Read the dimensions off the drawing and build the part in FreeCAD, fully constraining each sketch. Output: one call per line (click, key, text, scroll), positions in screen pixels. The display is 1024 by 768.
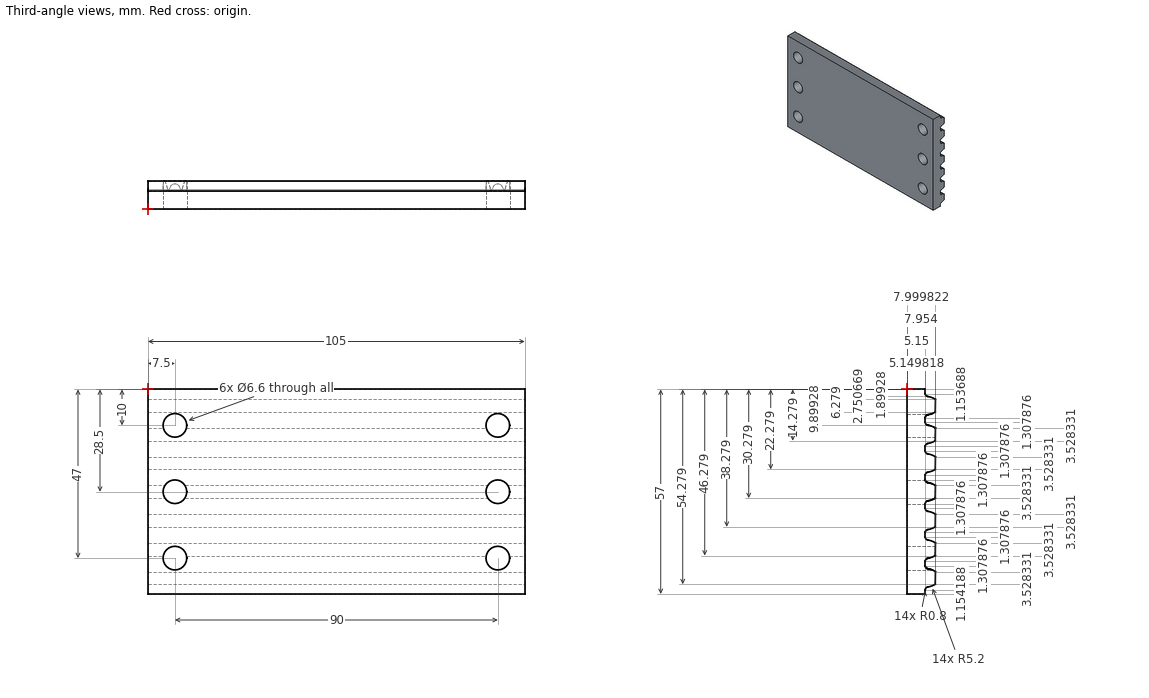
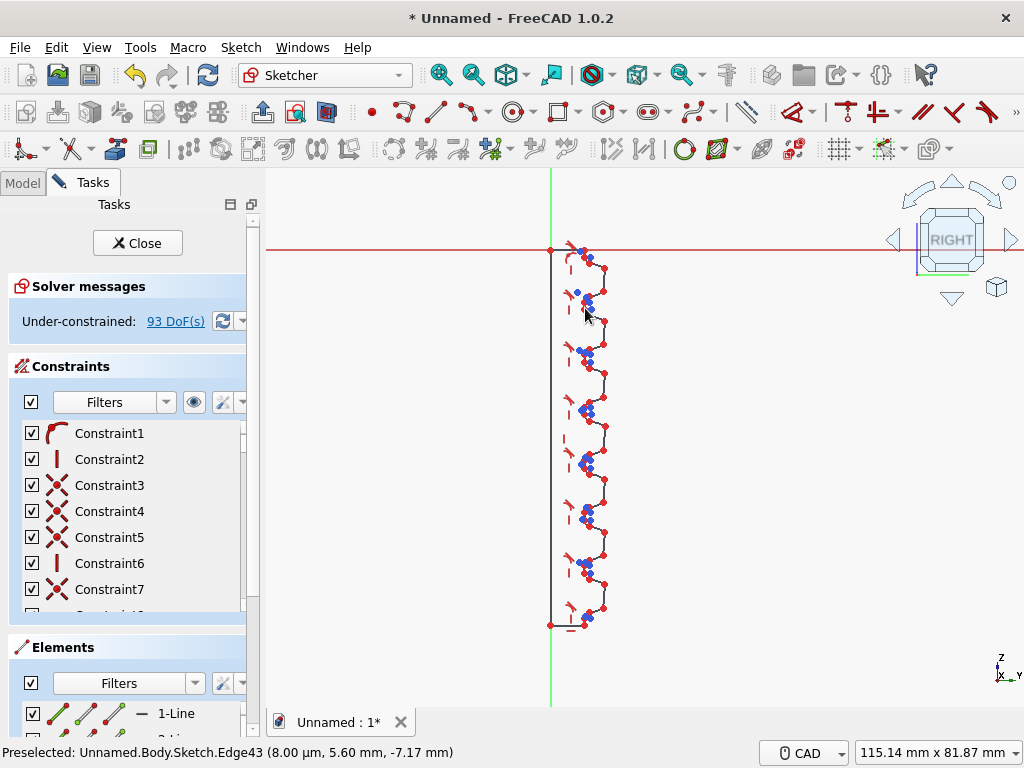
scroll(587, 614, up, 9)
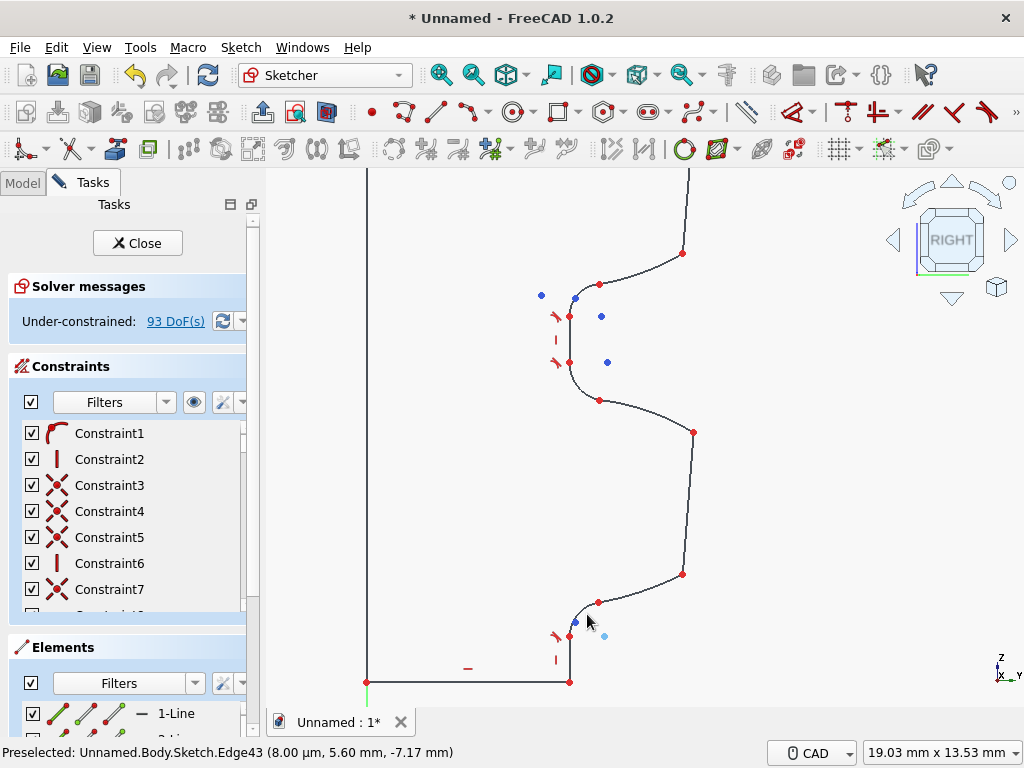
click(585, 608)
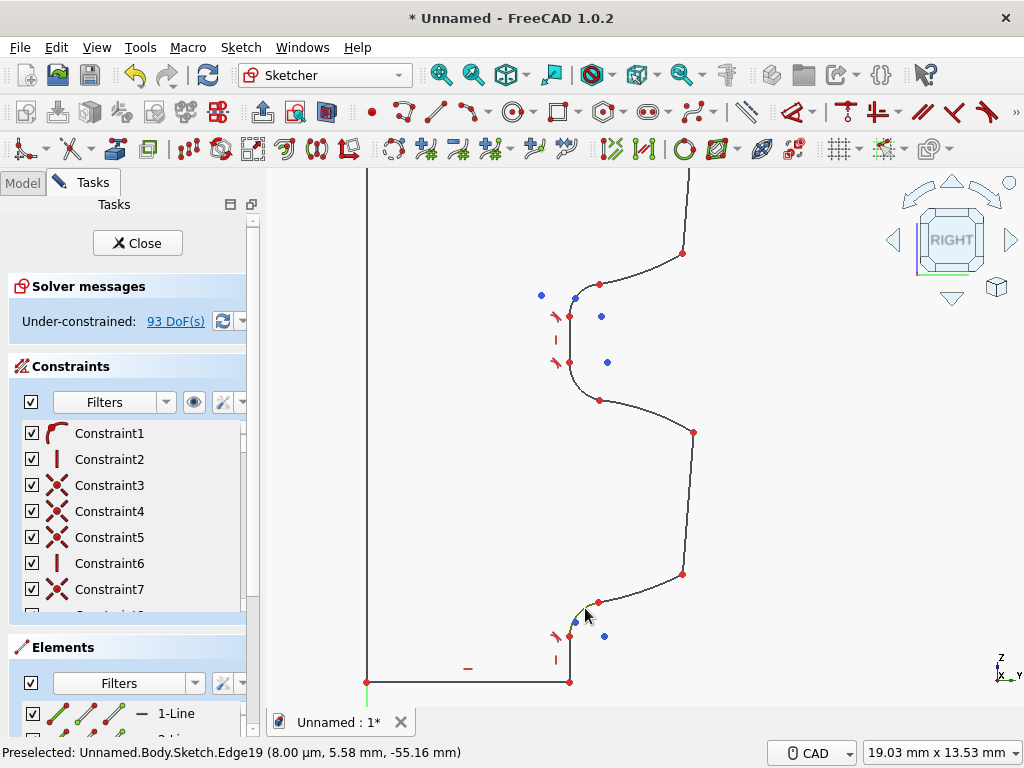
click(625, 597)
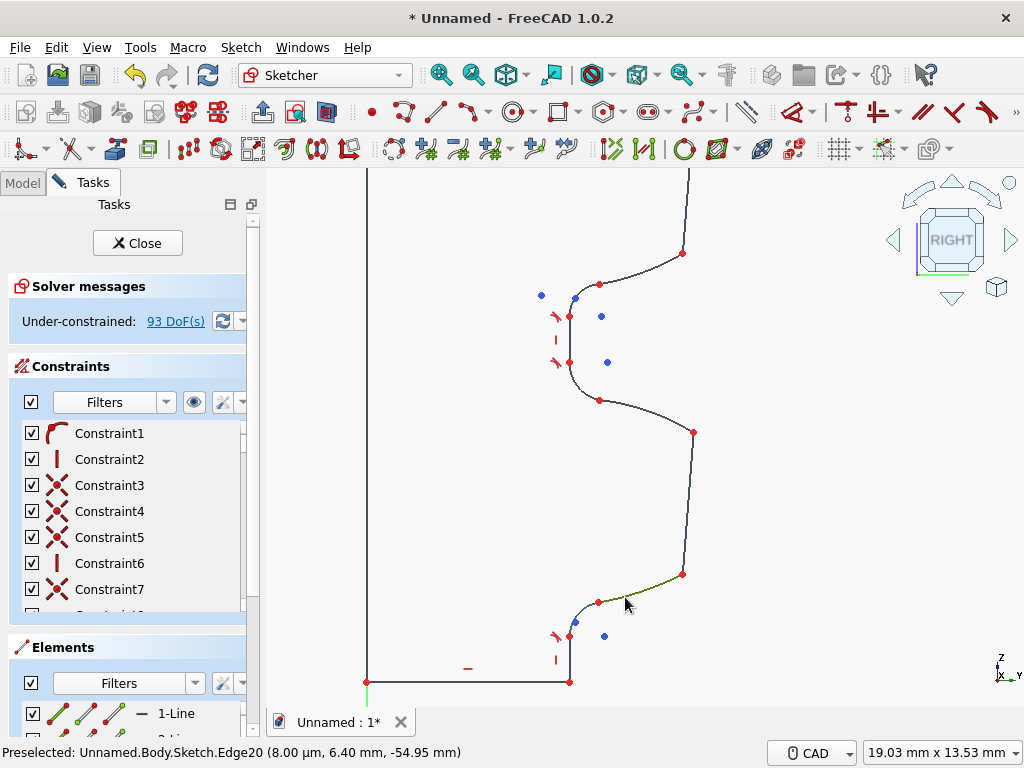
click(988, 112)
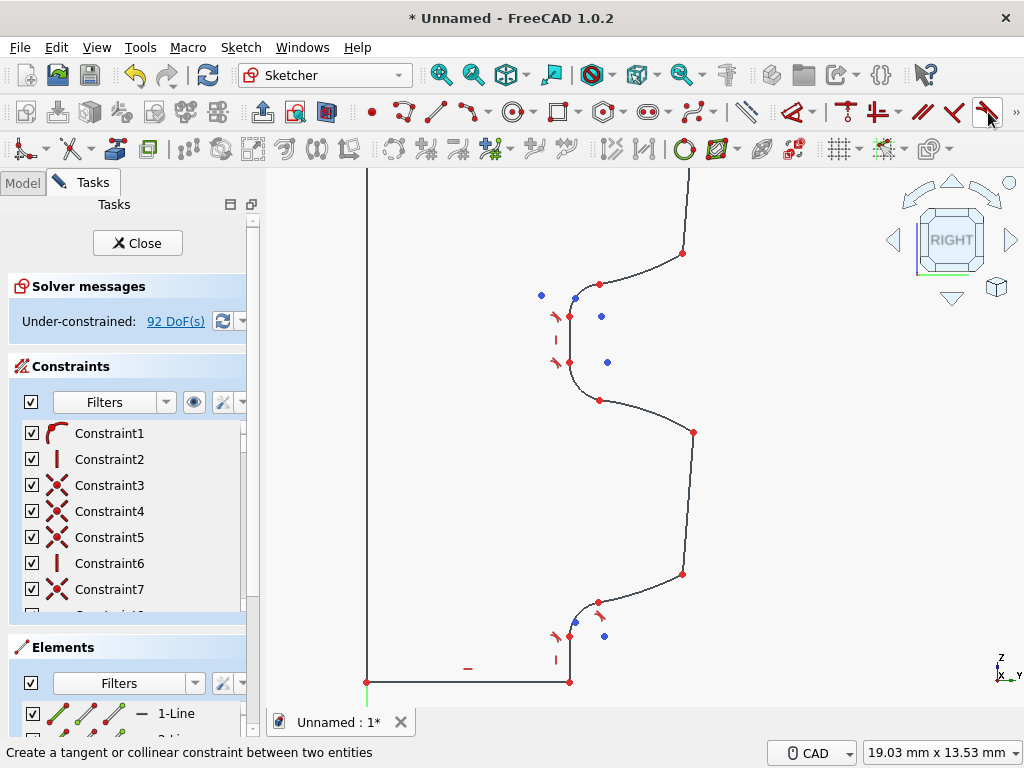
click(667, 419)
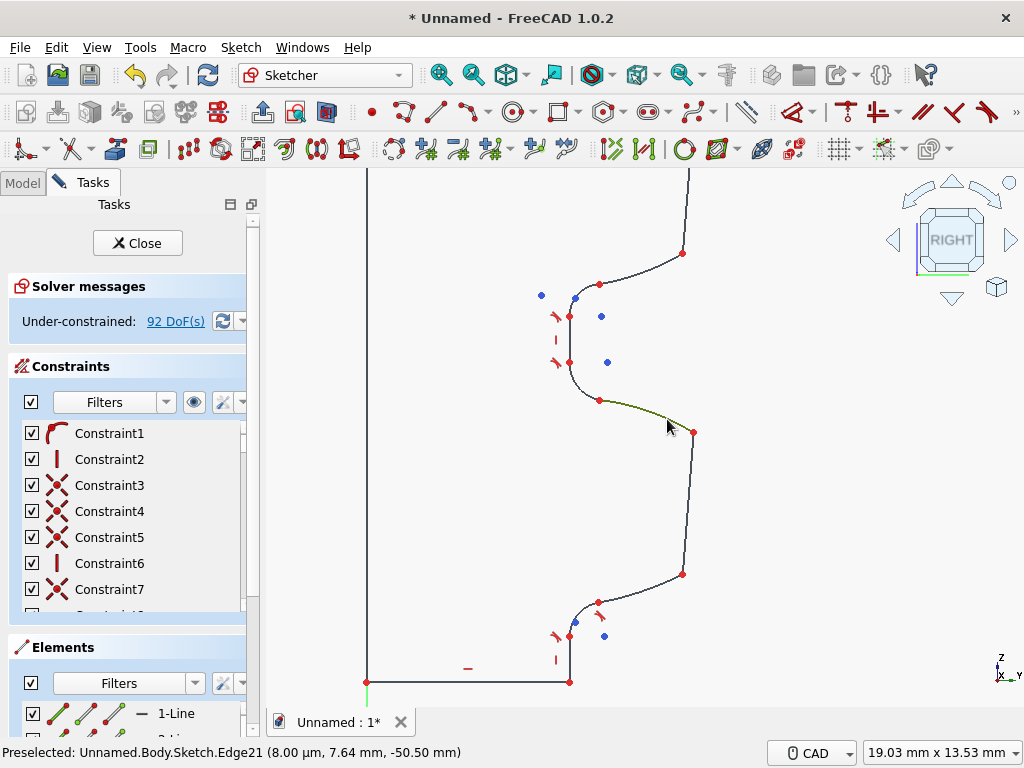
click(573, 378)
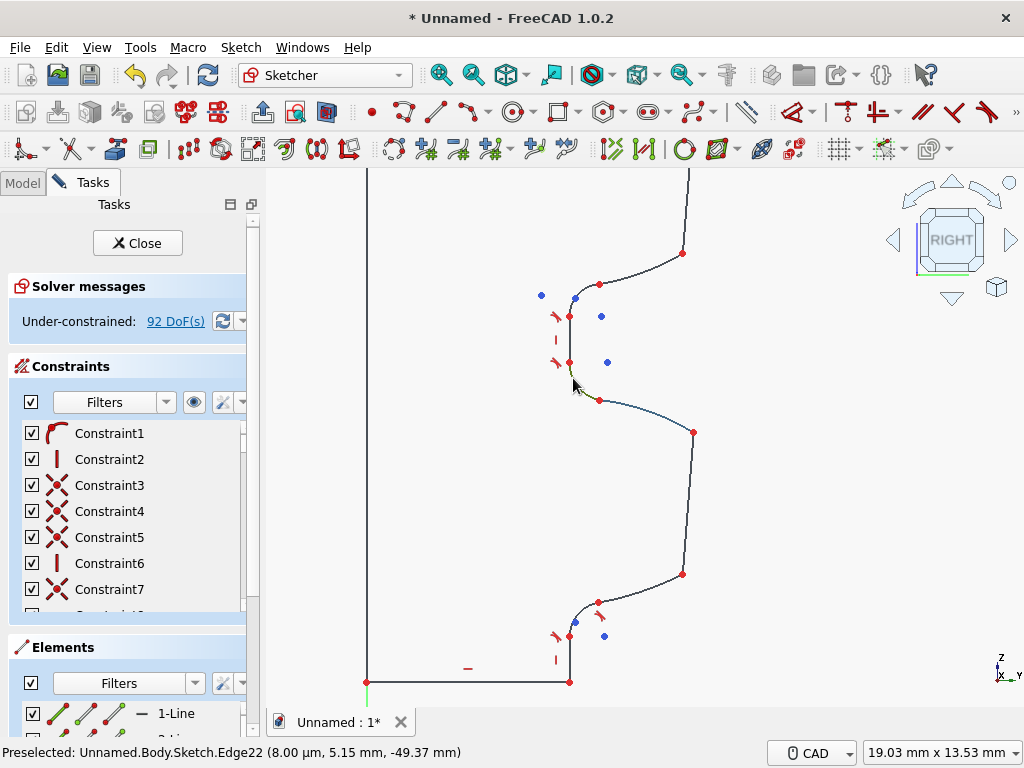
click(988, 112)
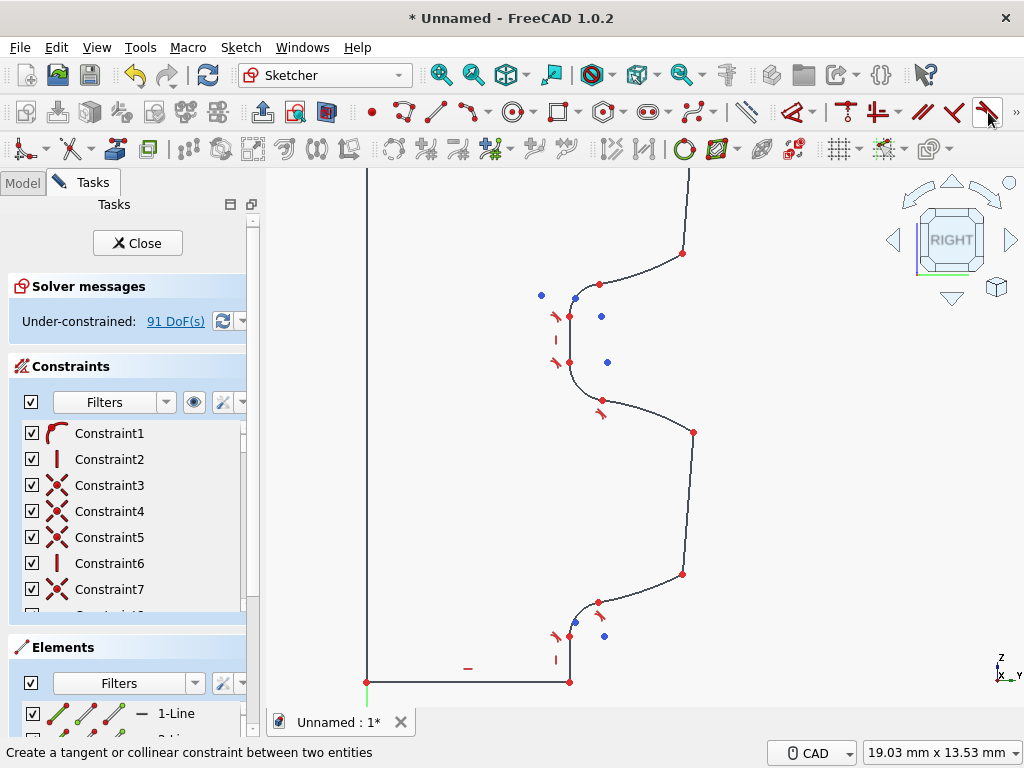
click(586, 288)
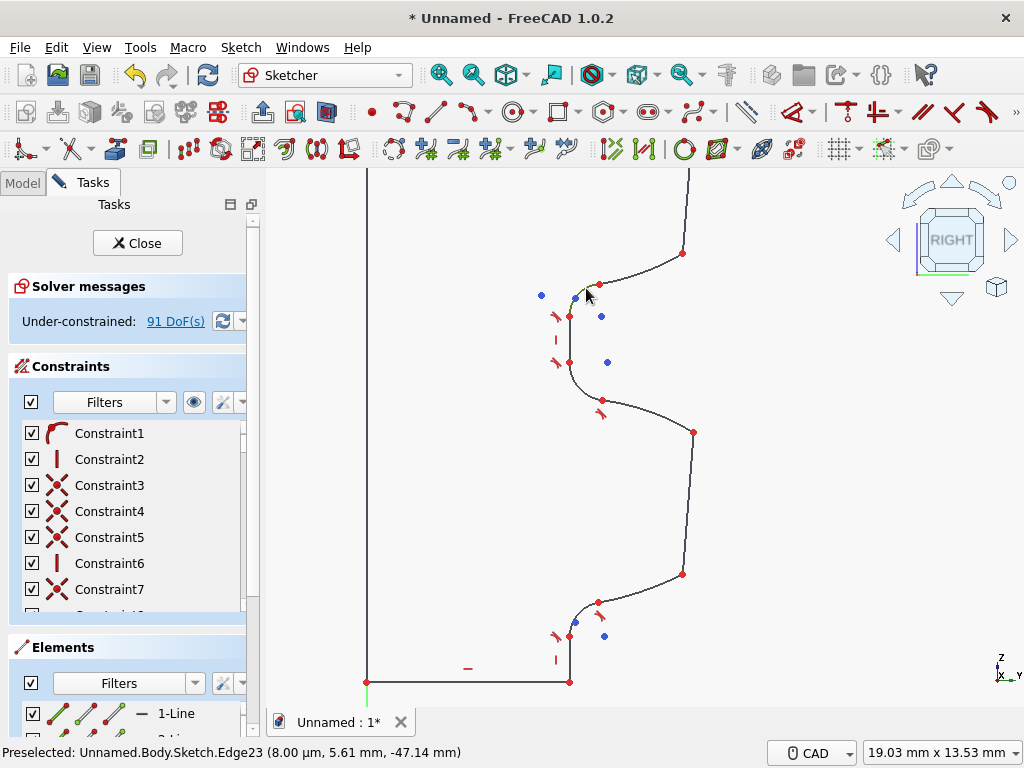
click(626, 278)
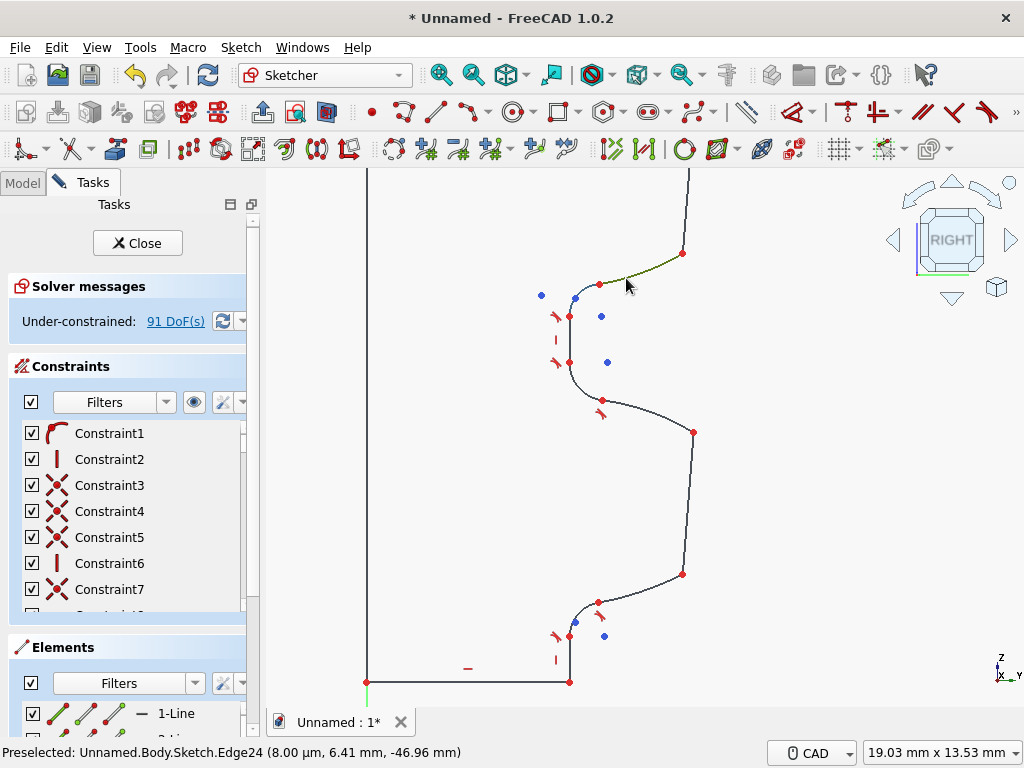
click(988, 112)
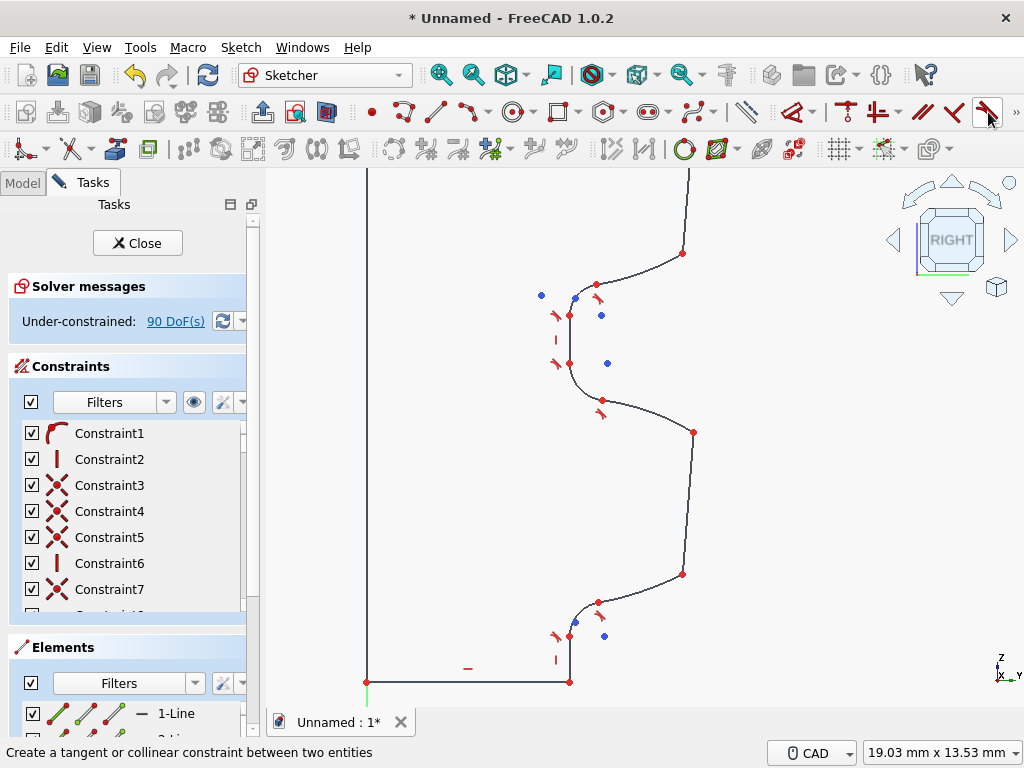
scroll(587, 614, down, 9)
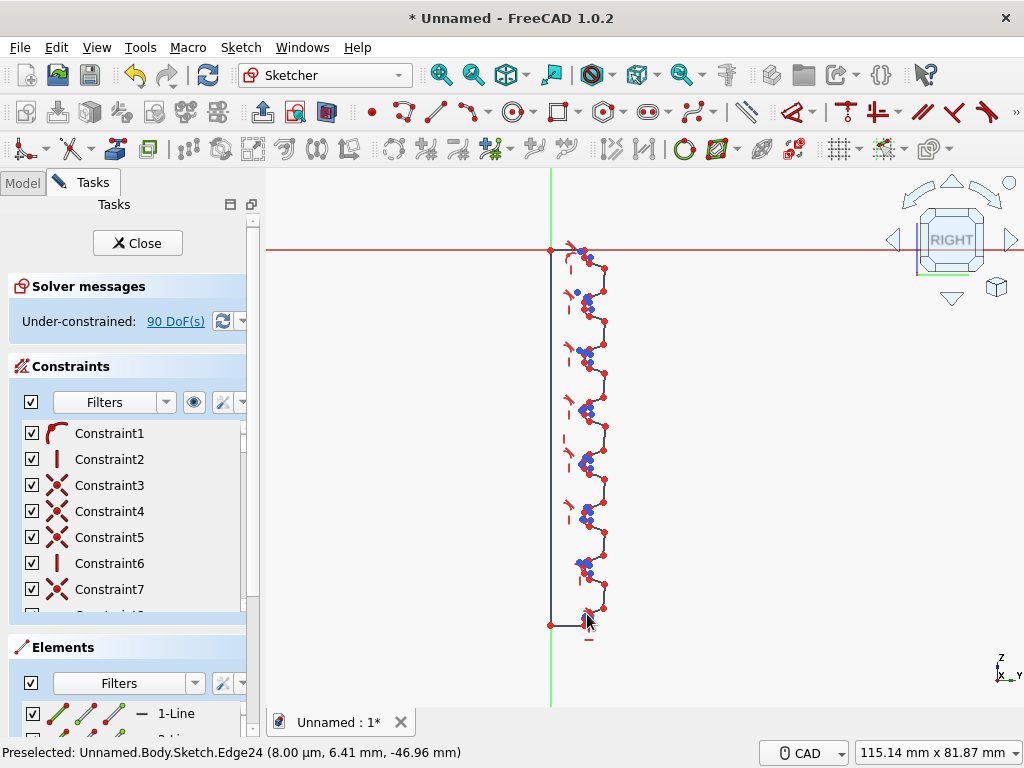
scroll(601, 530, up, 6)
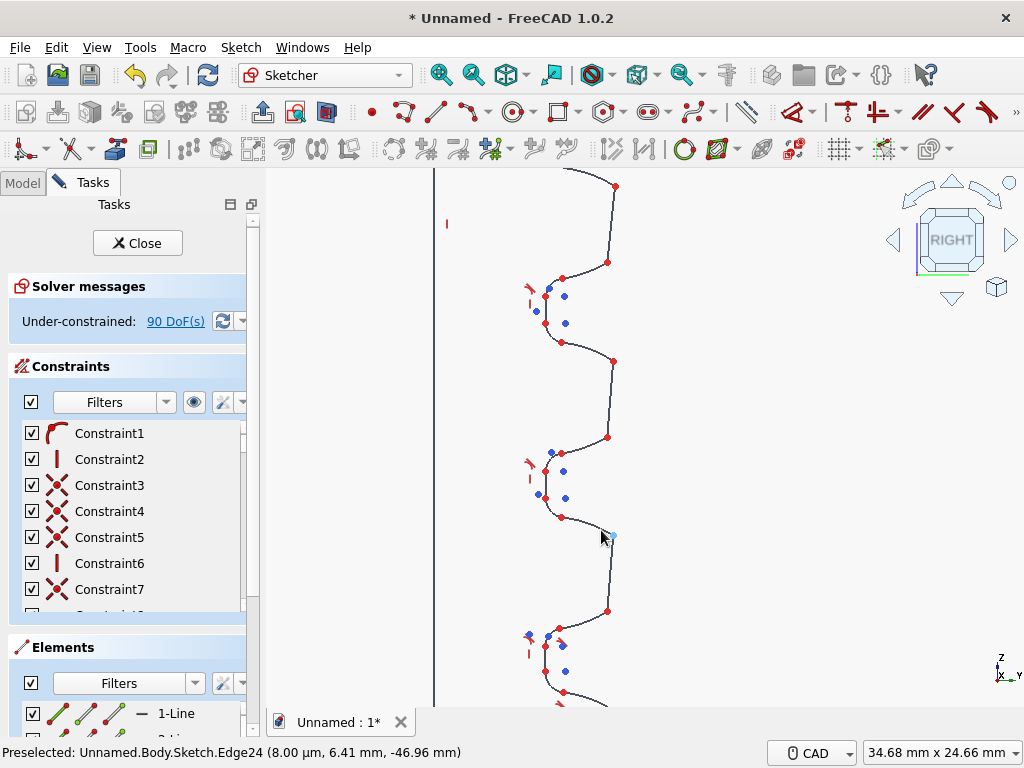
click(599, 528)